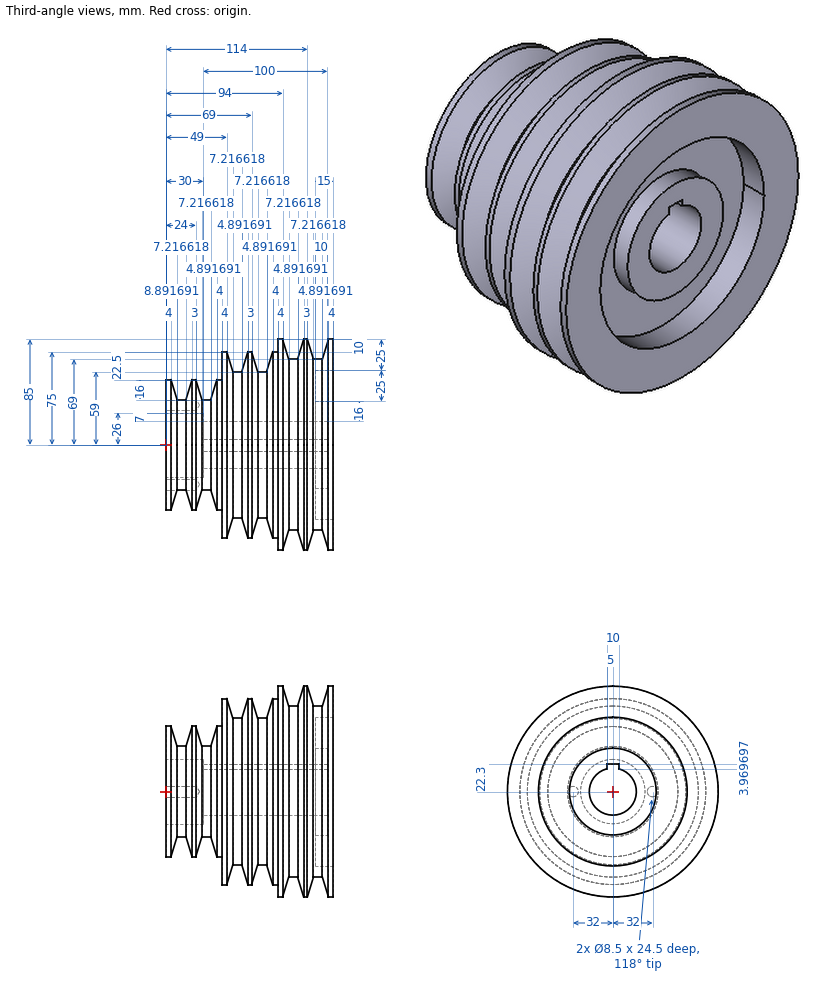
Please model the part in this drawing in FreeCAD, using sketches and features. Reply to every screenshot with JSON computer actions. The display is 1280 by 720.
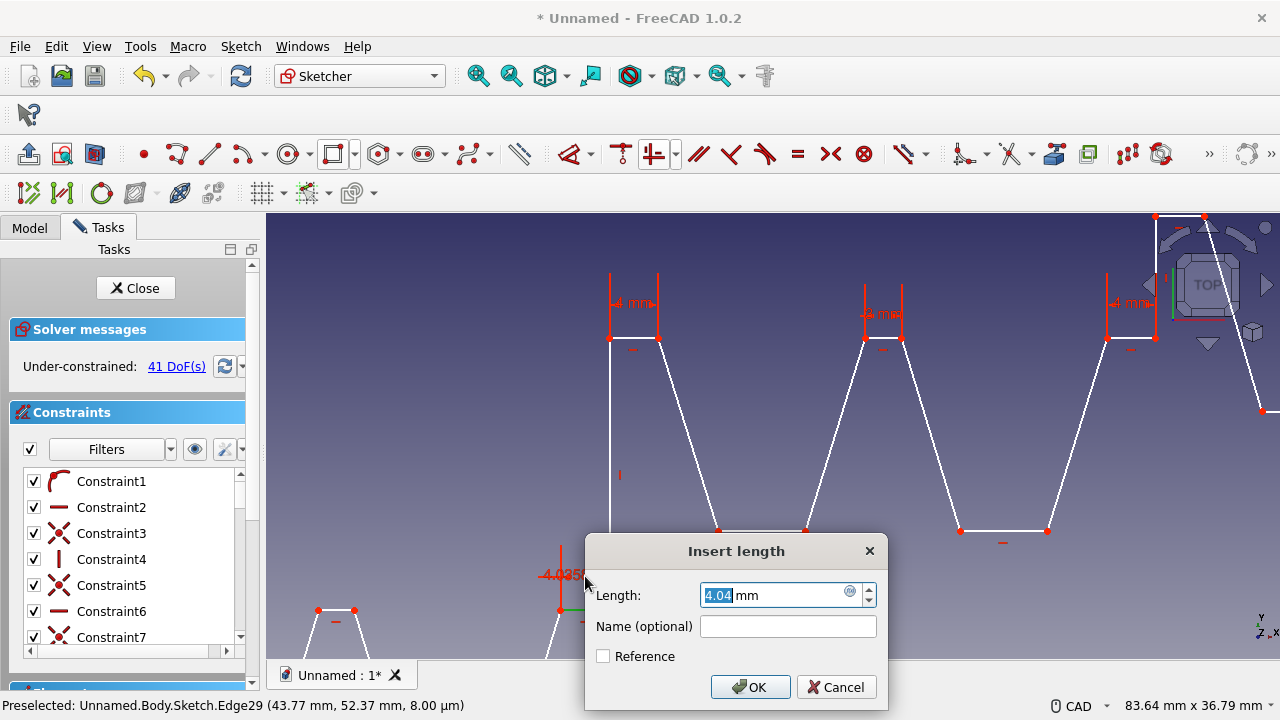
{"action": "type", "text": "4"}
{"action": "key", "text": "Return"}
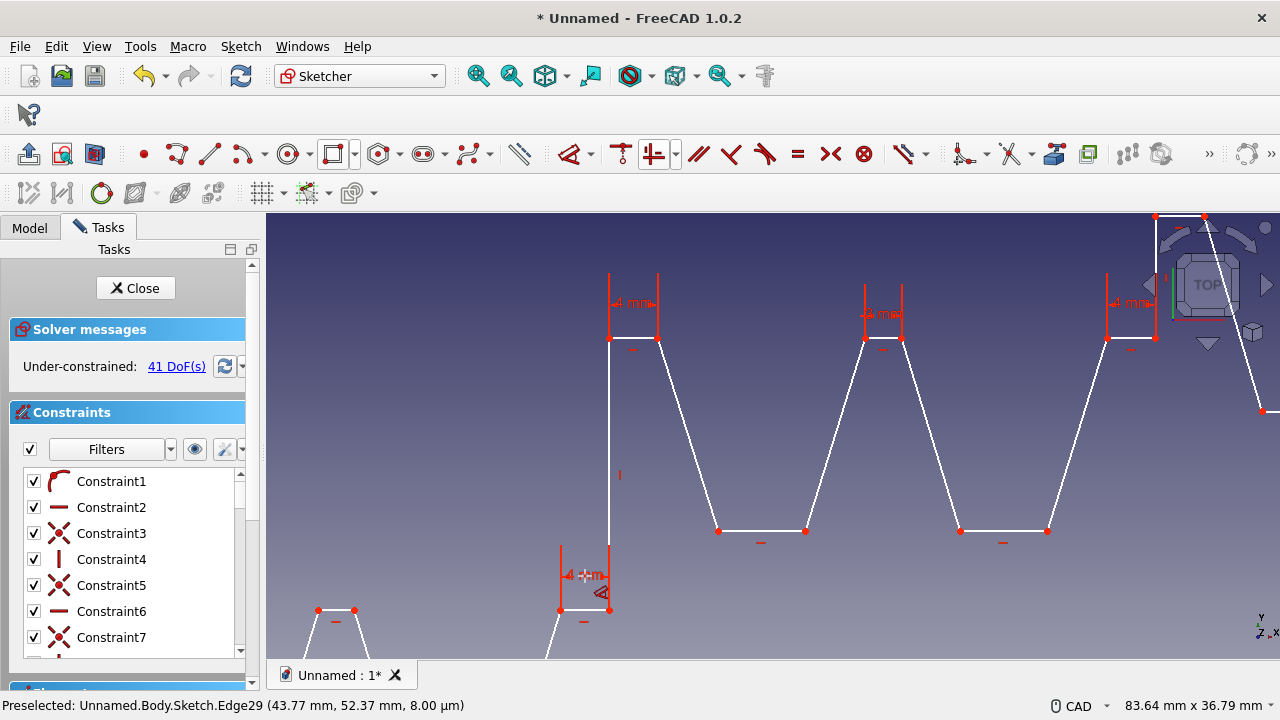
{"action": "scroll", "coordinate": [344, 610], "scroll_direction": "up", "scroll_amount": 2}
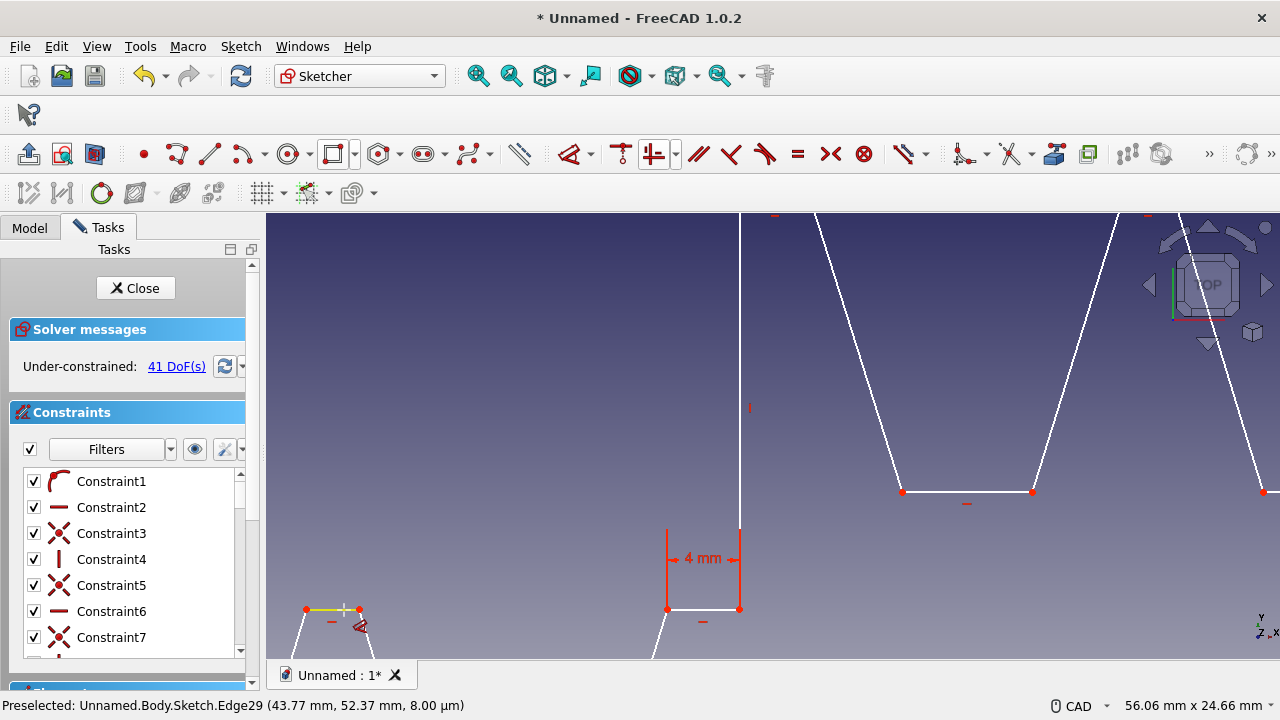
{"action": "left_click", "coordinate": [343, 610]}
{"action": "left_click", "coordinate": [333, 576]}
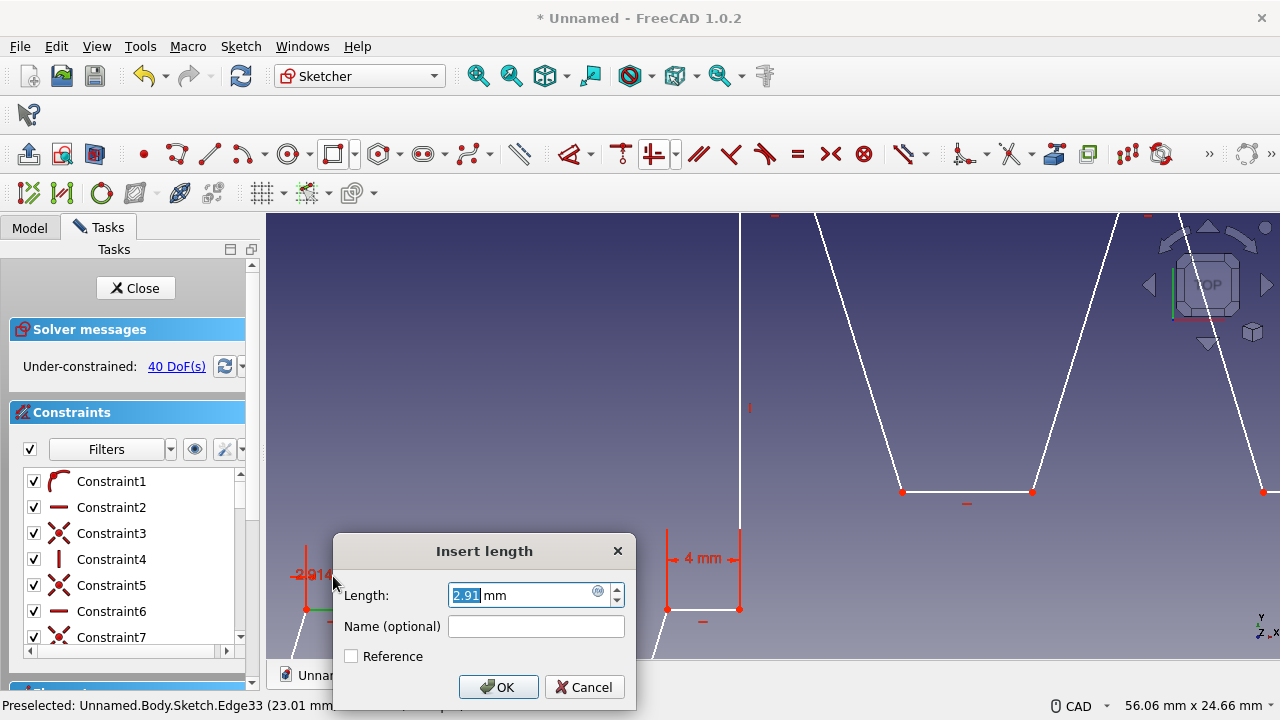
{"action": "type", "text": "3"}
{"action": "key", "text": "Return"}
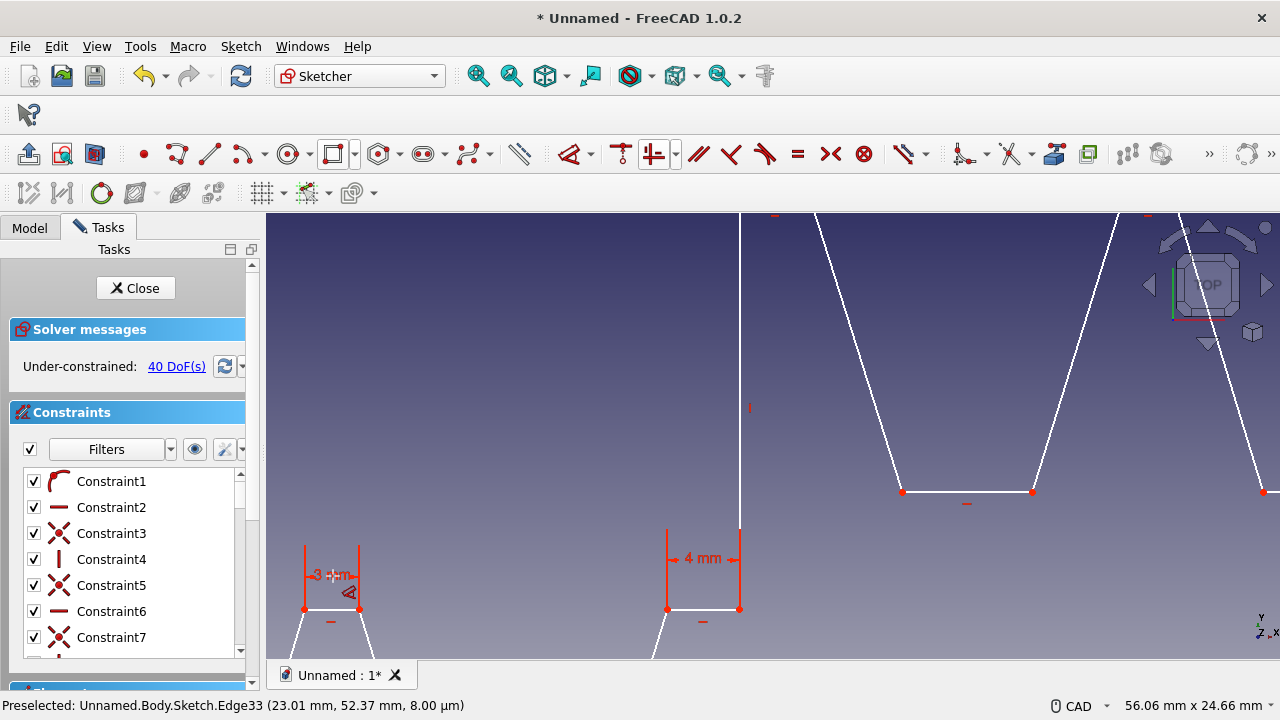
{"action": "scroll", "coordinate": [617, 366], "scroll_direction": "down", "scroll_amount": 9}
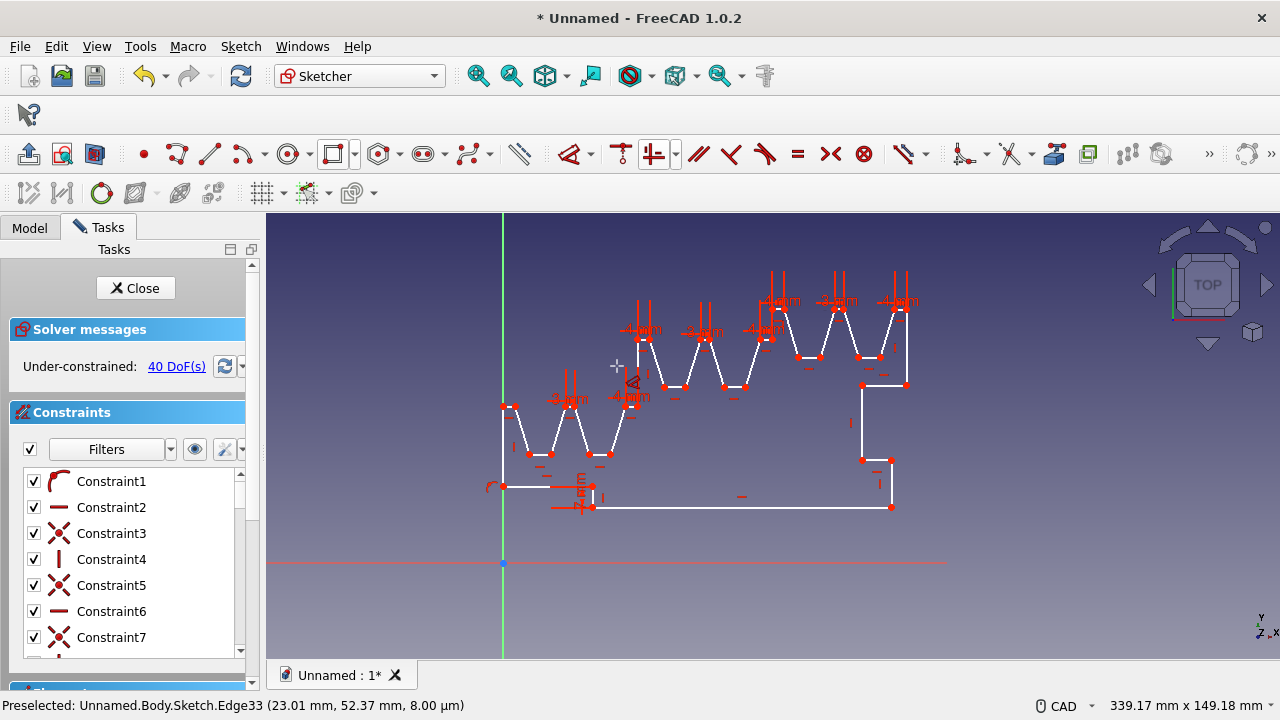
{"action": "scroll", "coordinate": [511, 407], "scroll_direction": "up", "scroll_amount": 7}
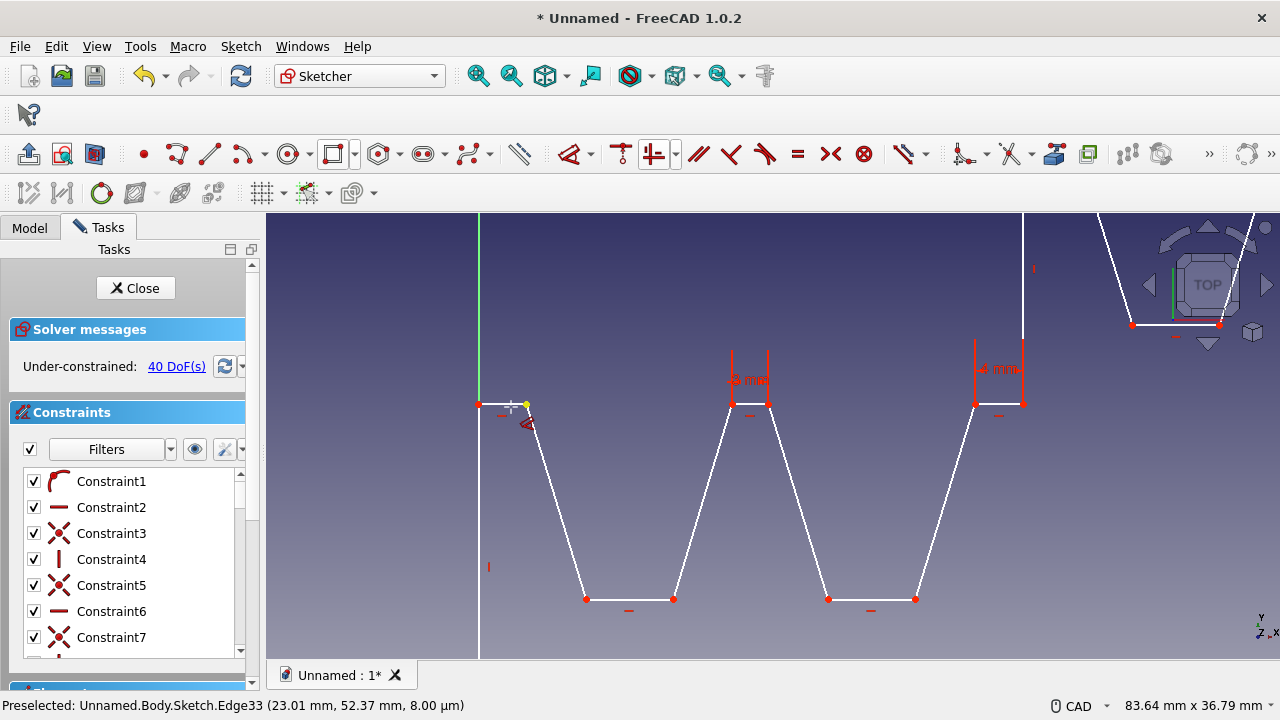
{"action": "left_click", "coordinate": [512, 404]}
{"action": "left_click", "coordinate": [503, 370]}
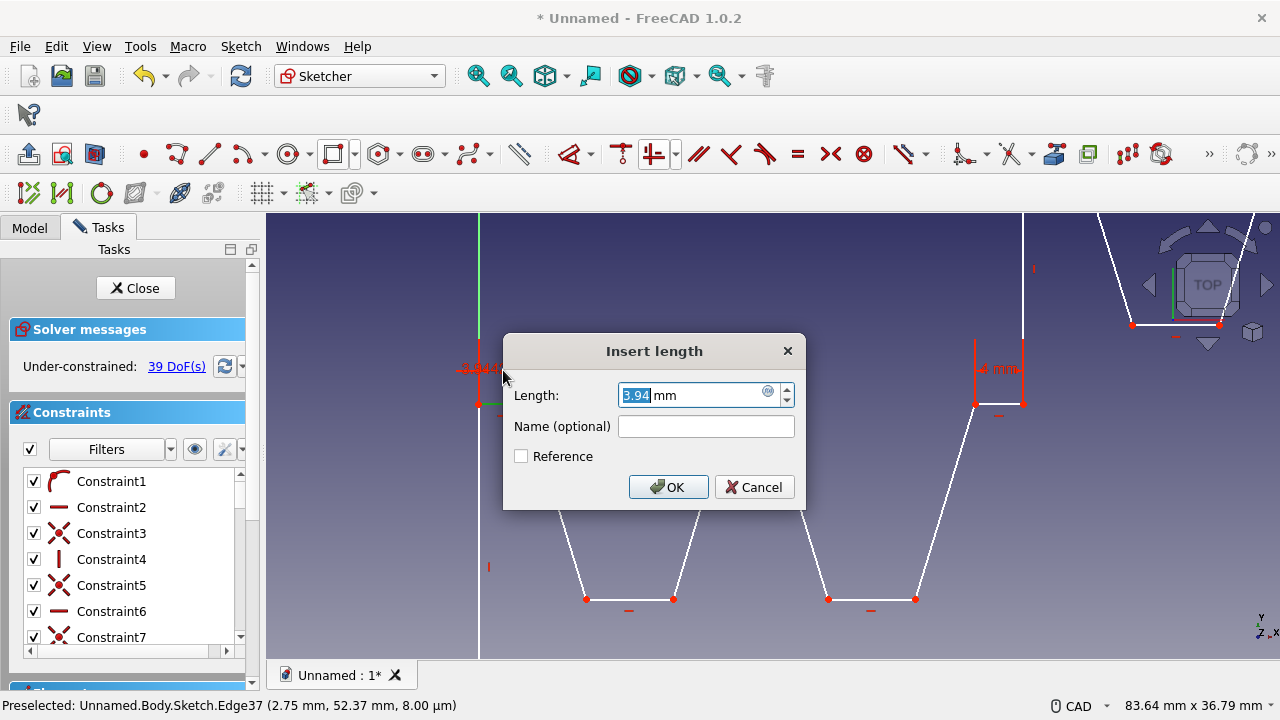
{"action": "type", "text": "4"}
{"action": "key", "text": "Return"}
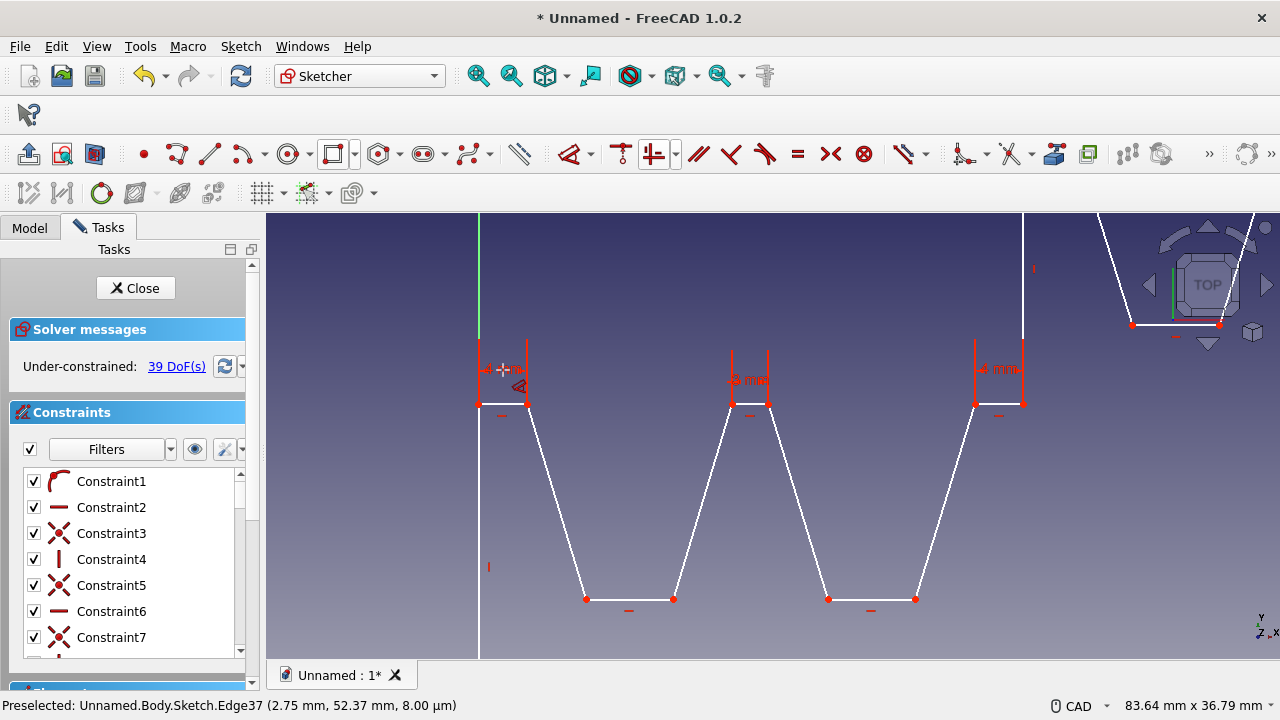
{"action": "scroll", "coordinate": [511, 407], "scroll_direction": "down", "scroll_amount": 7}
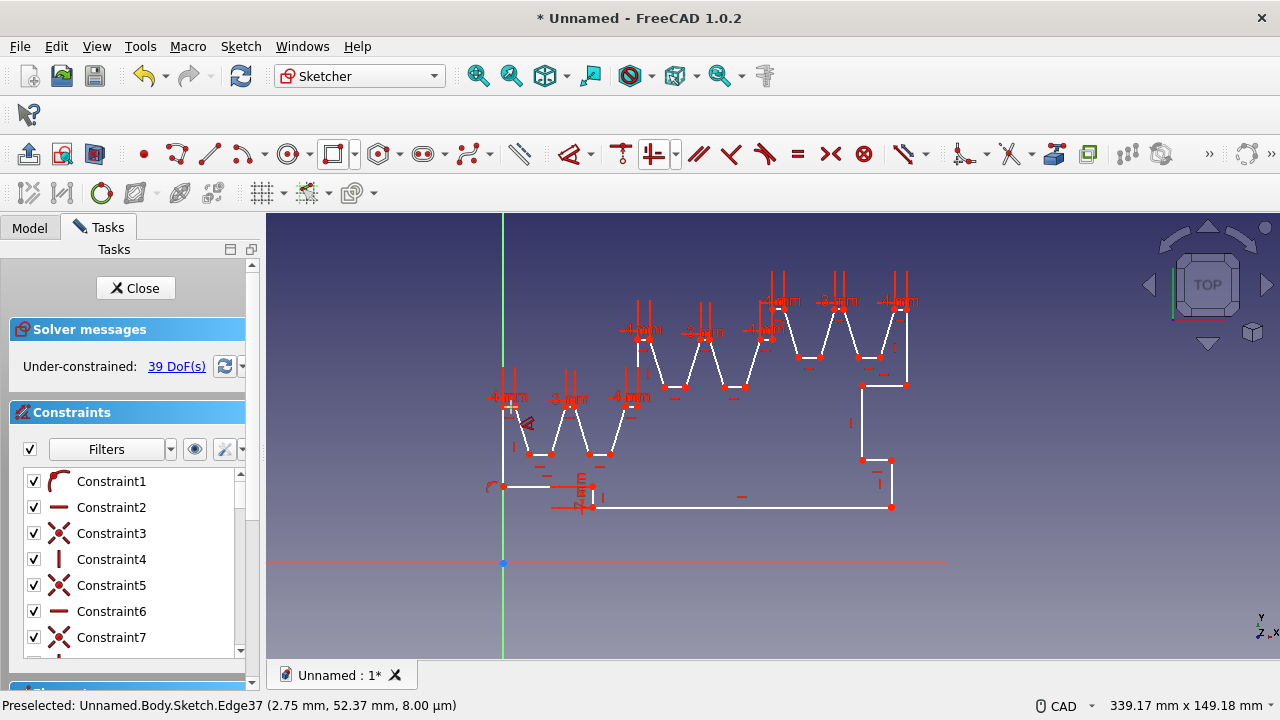
{"action": "left_click", "coordinate": [530, 487]}
{"action": "left_click", "coordinate": [548, 521]}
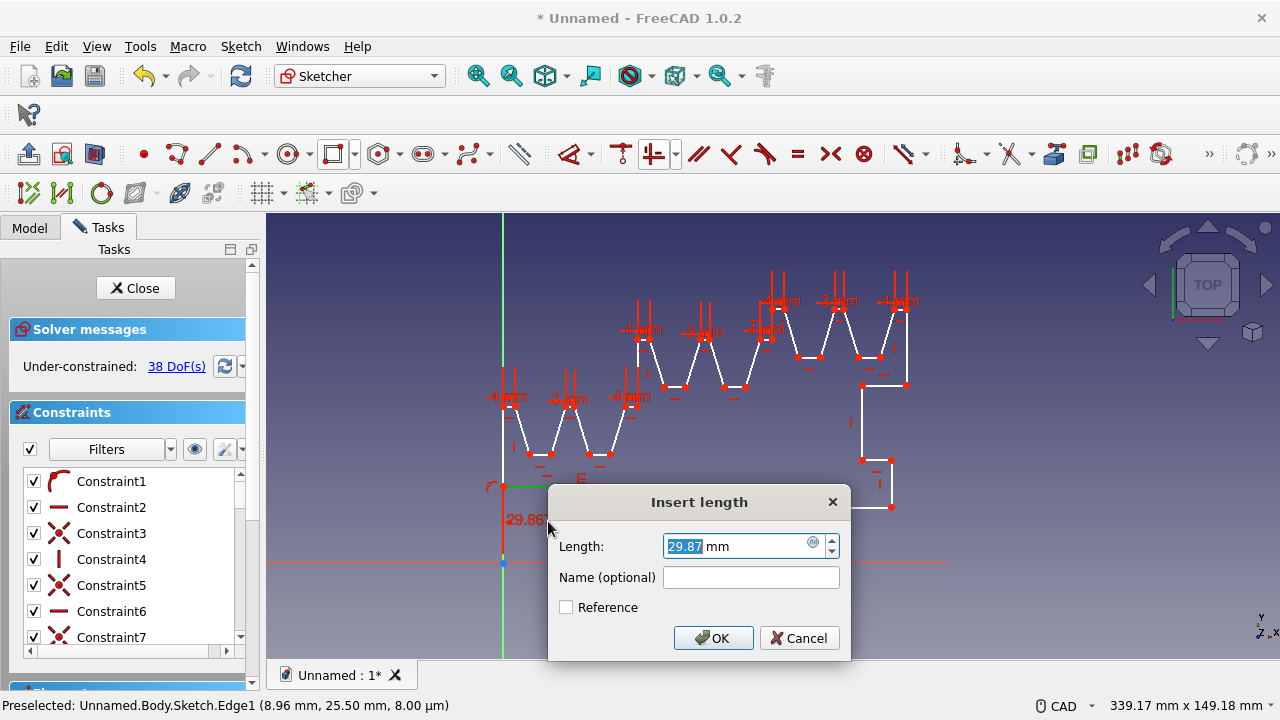
{"action": "type", "text": "30"}
{"action": "key", "text": "Return"}